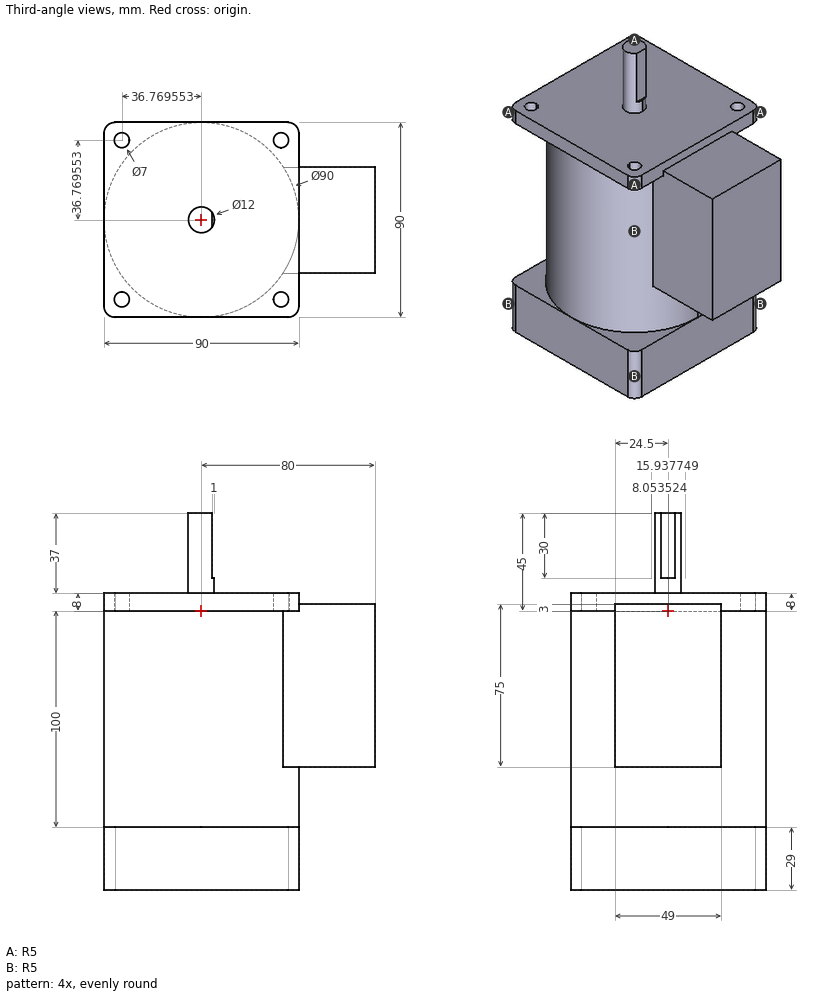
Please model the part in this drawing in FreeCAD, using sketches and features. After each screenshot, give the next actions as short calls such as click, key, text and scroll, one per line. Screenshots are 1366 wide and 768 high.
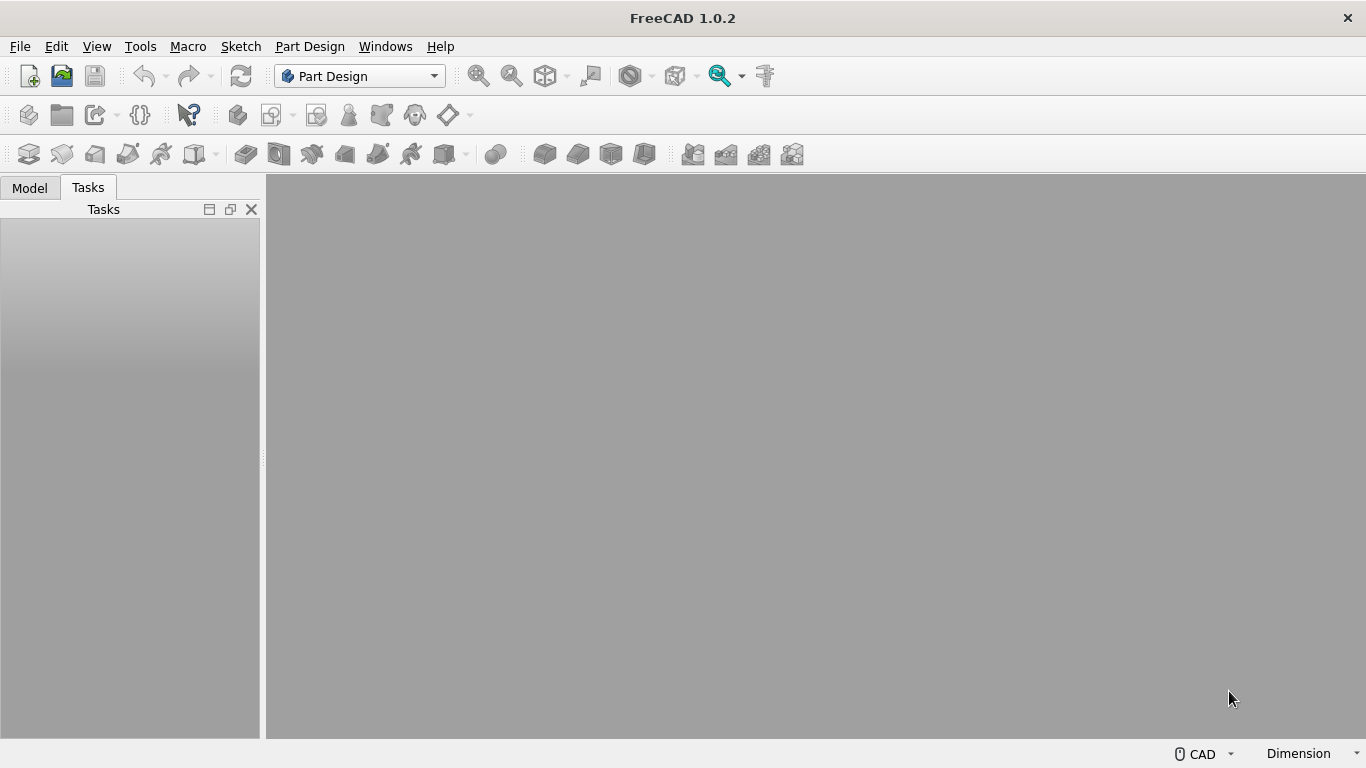
click(29, 76)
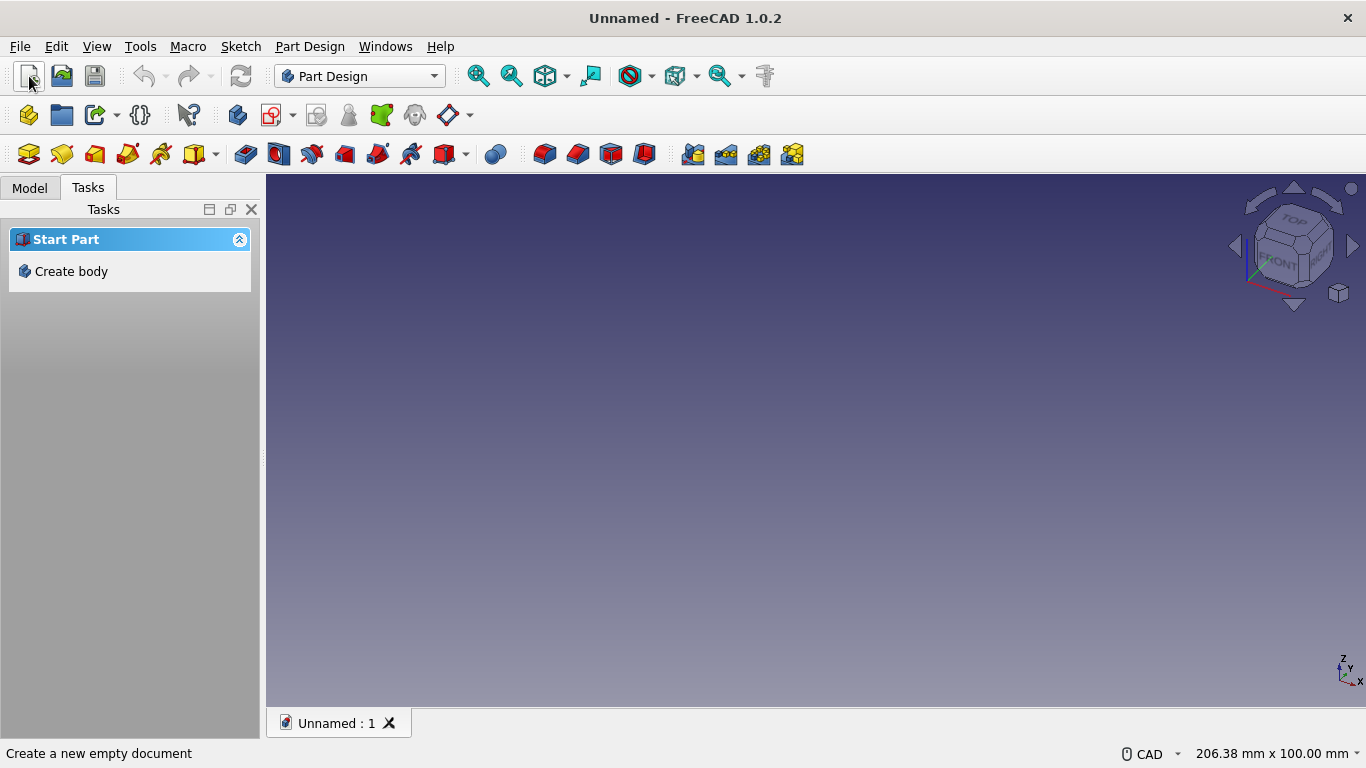
click(270, 116)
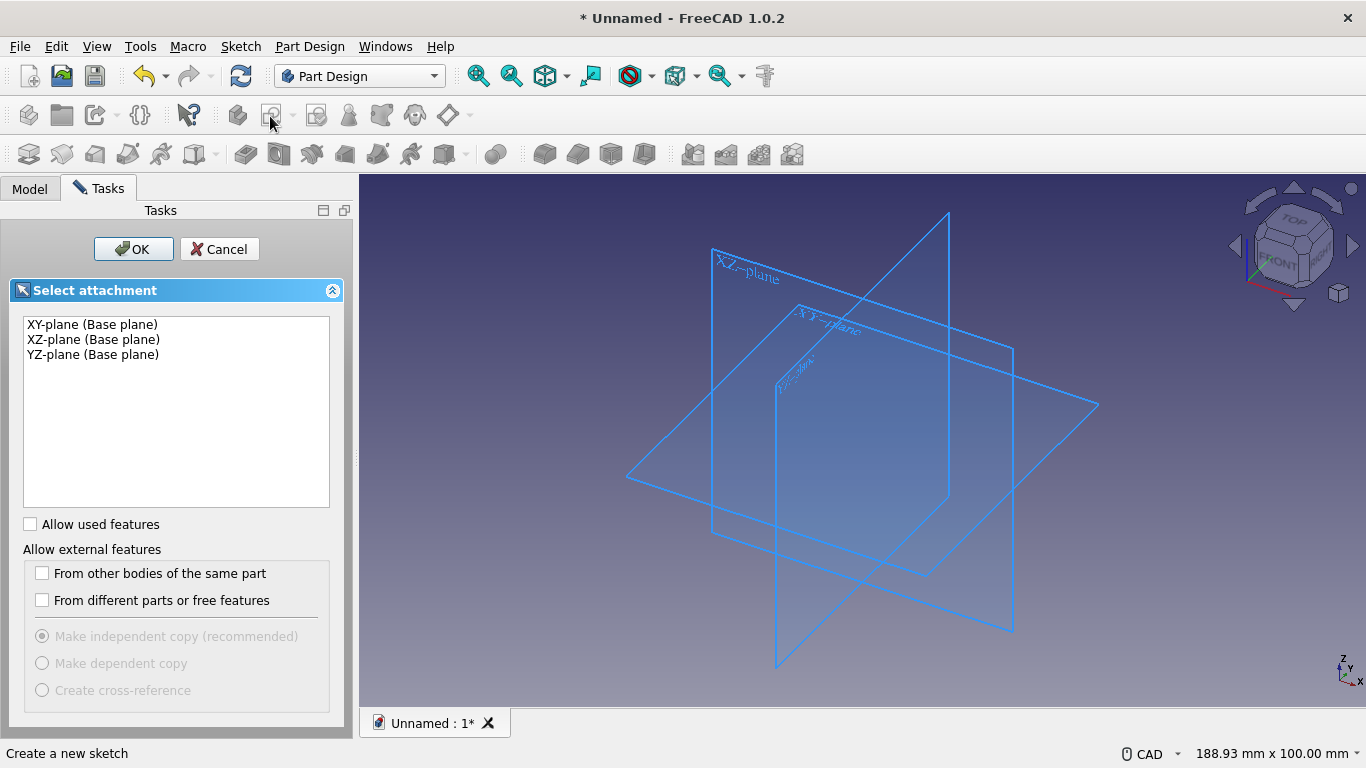
click(84, 324)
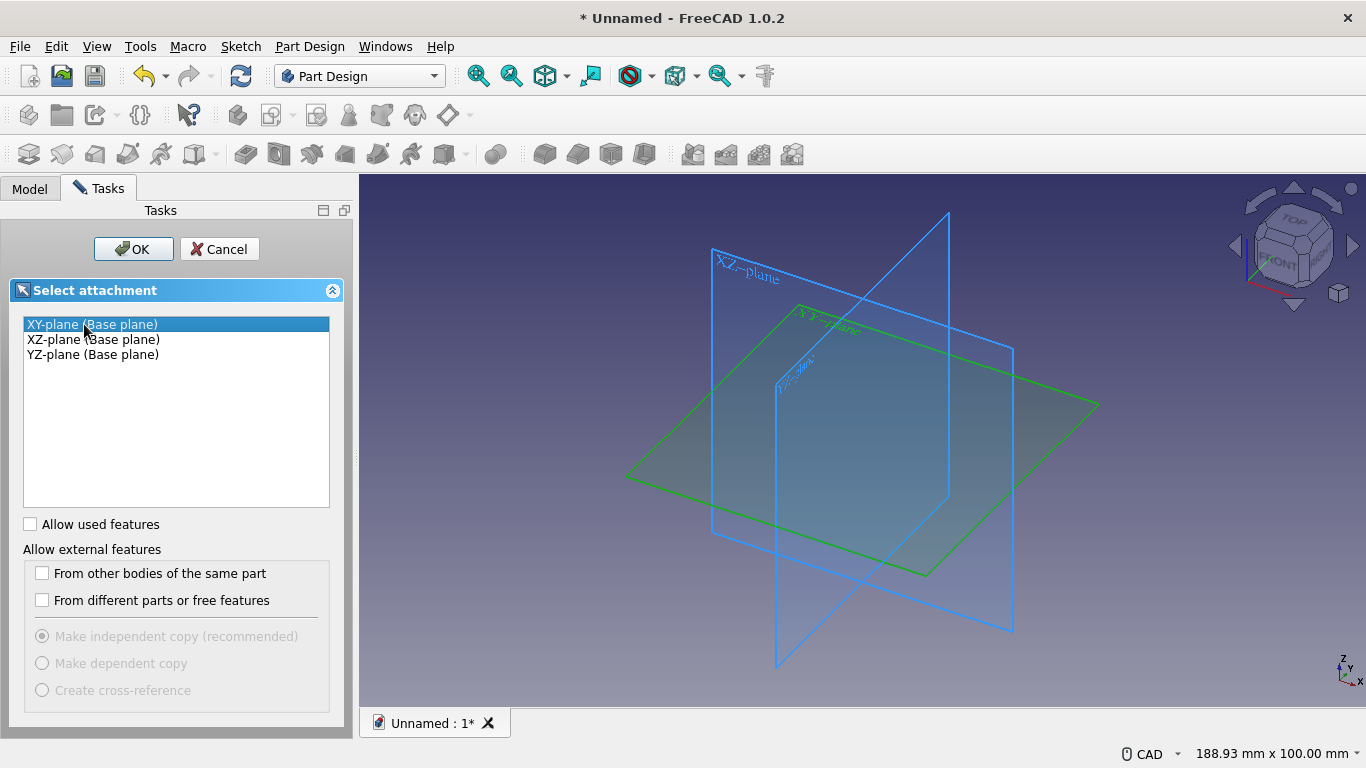
click(134, 249)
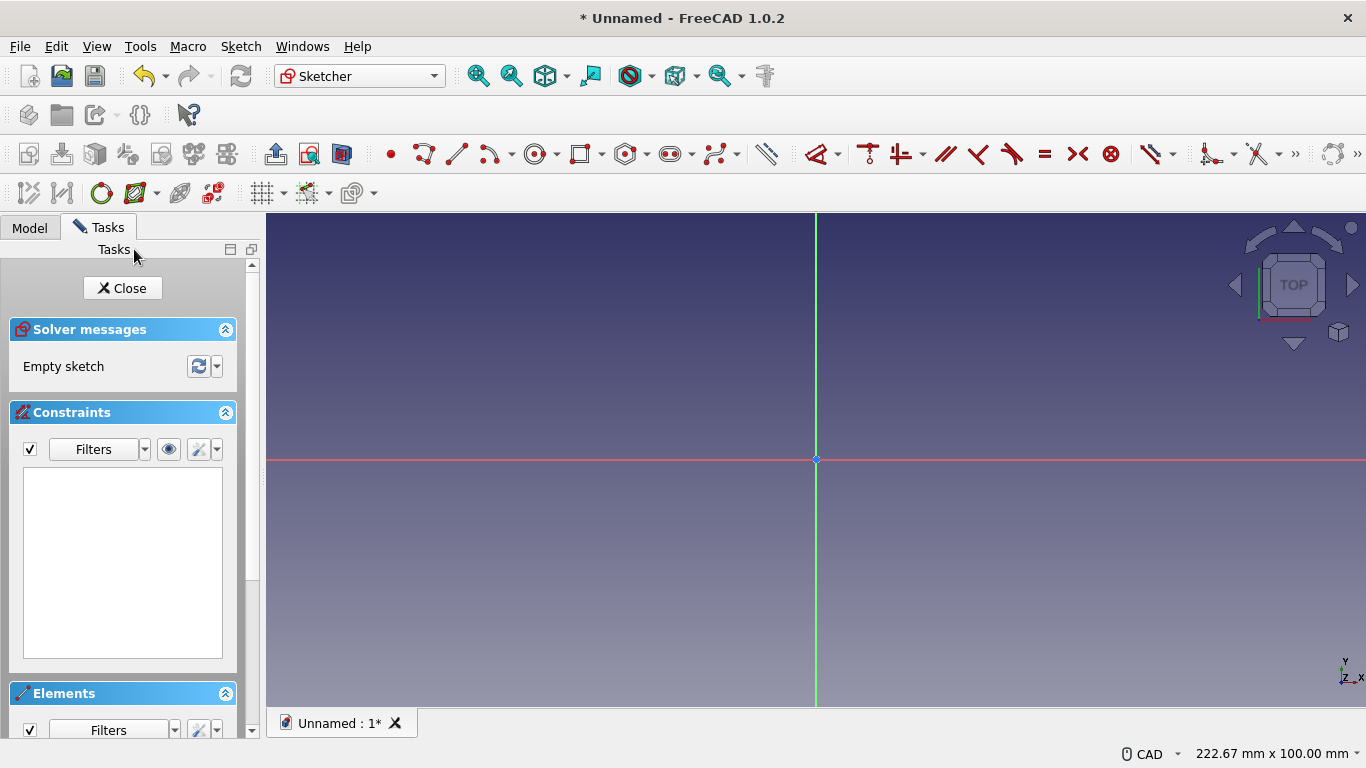
scroll(608, 460, down, 2)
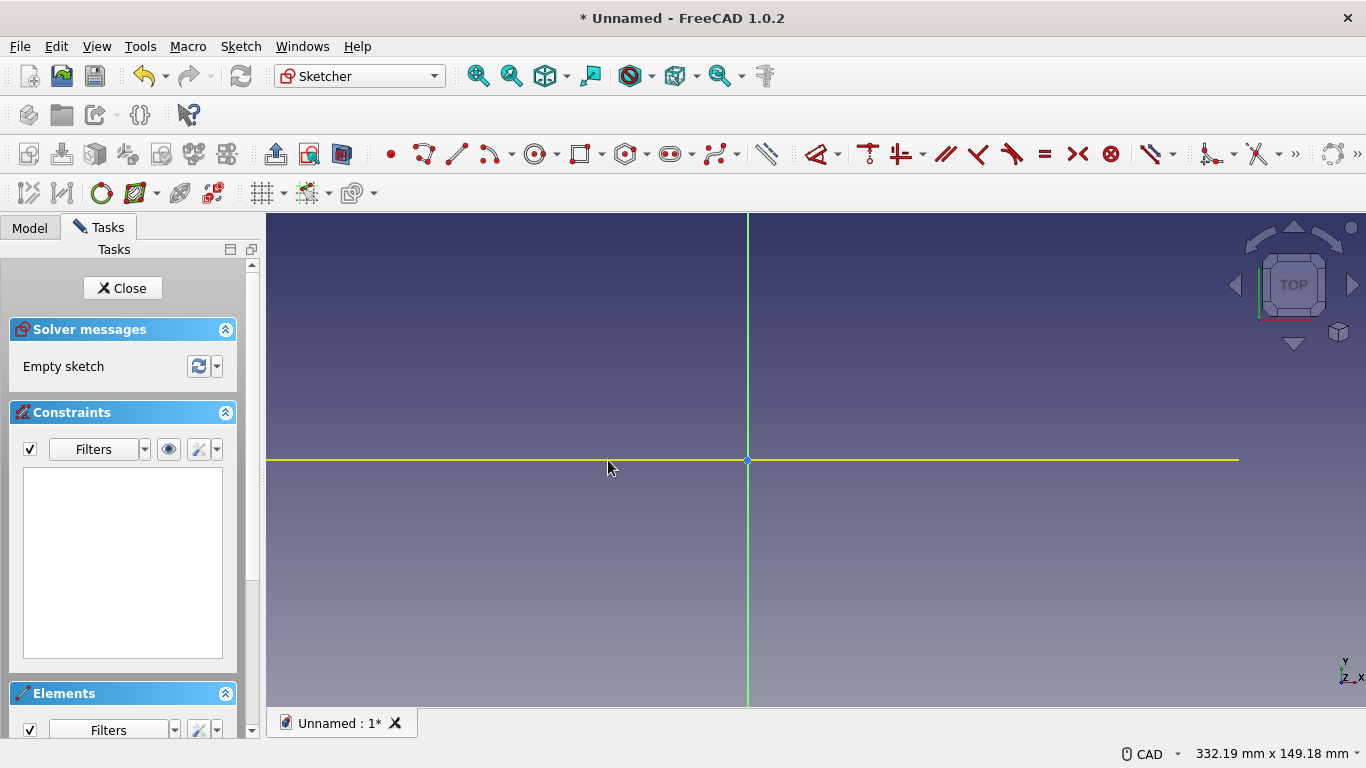
key(g)
key(v)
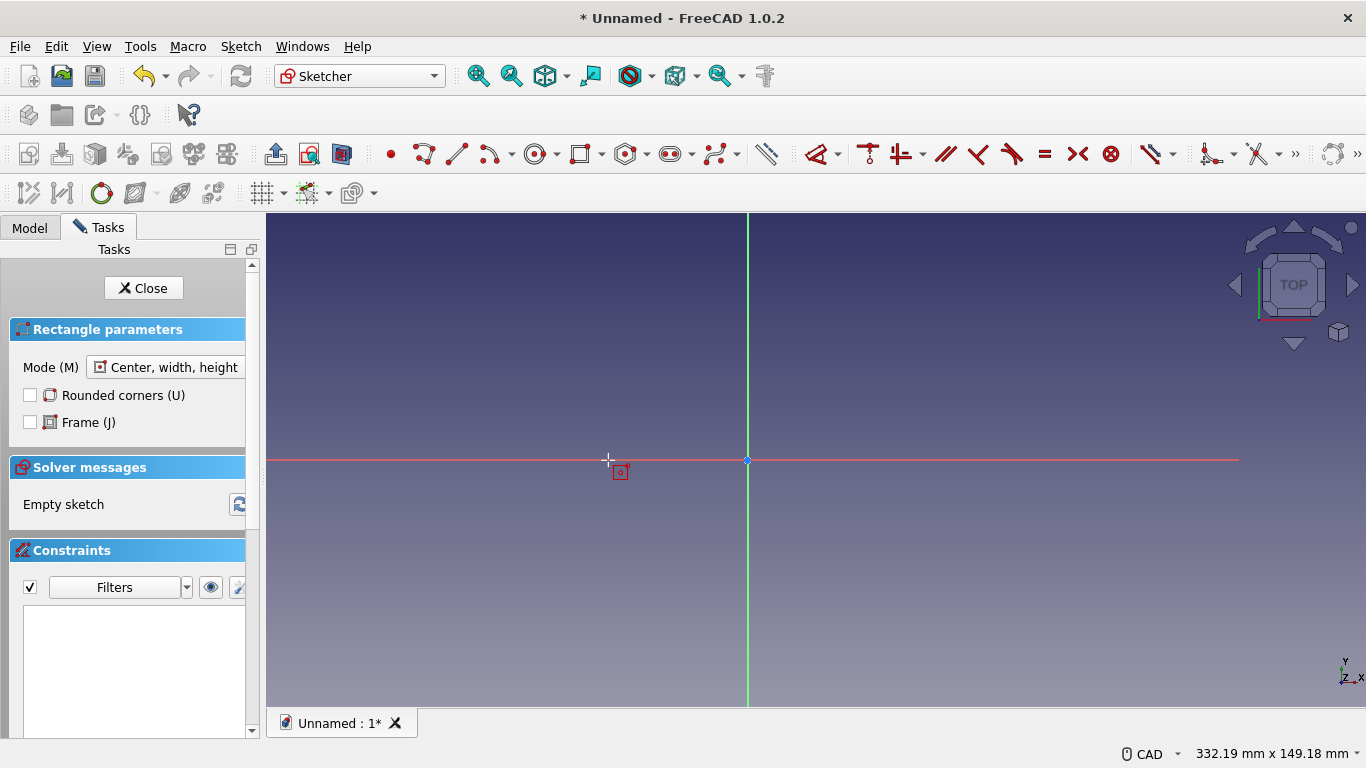
click(748, 460)
click(897, 311)
key(Escape)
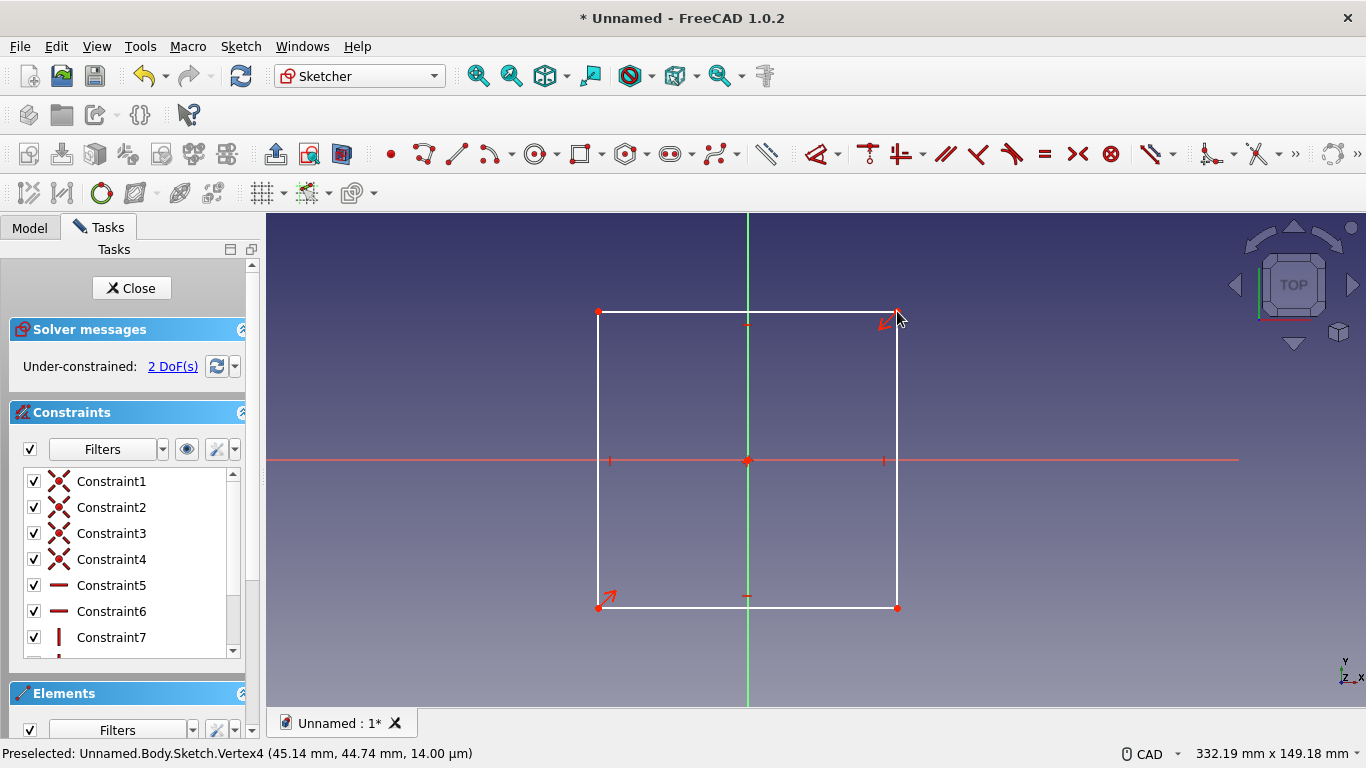
click(688, 608)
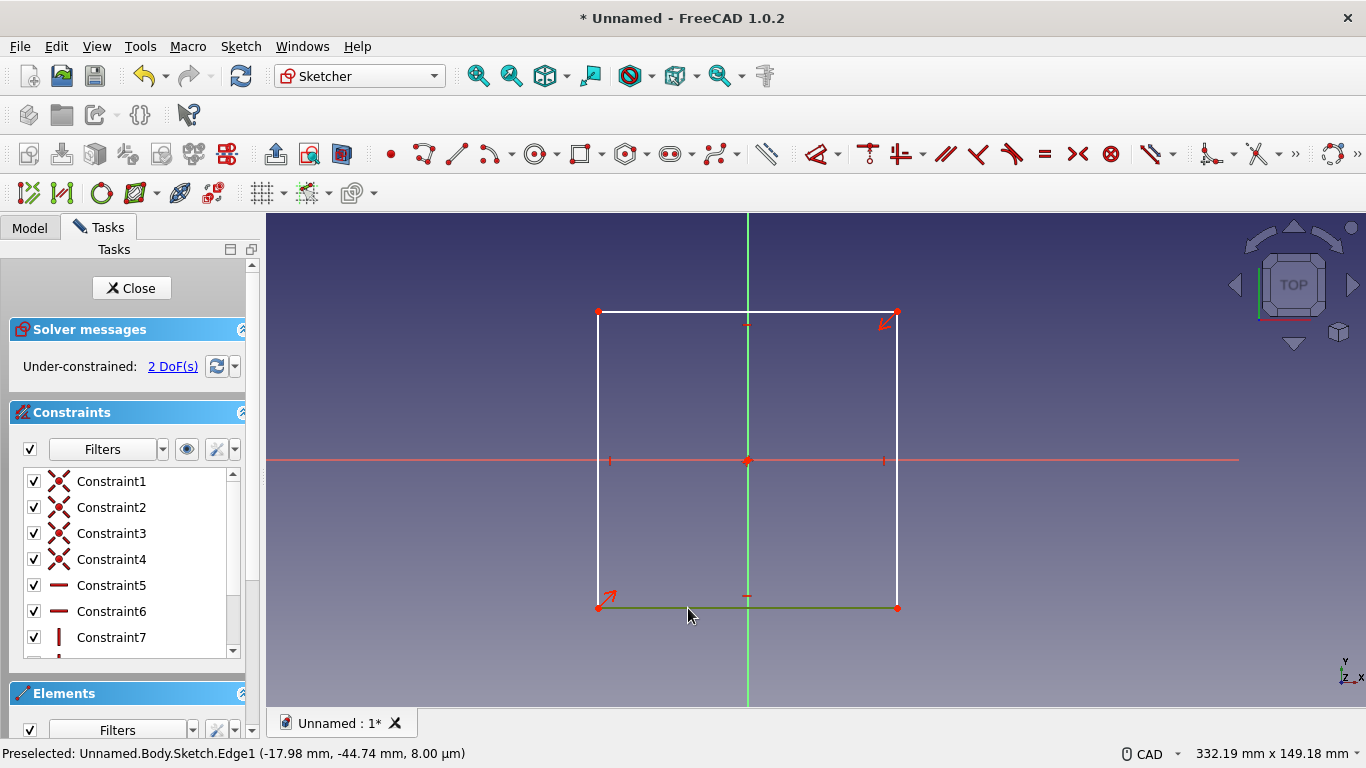
click(838, 154)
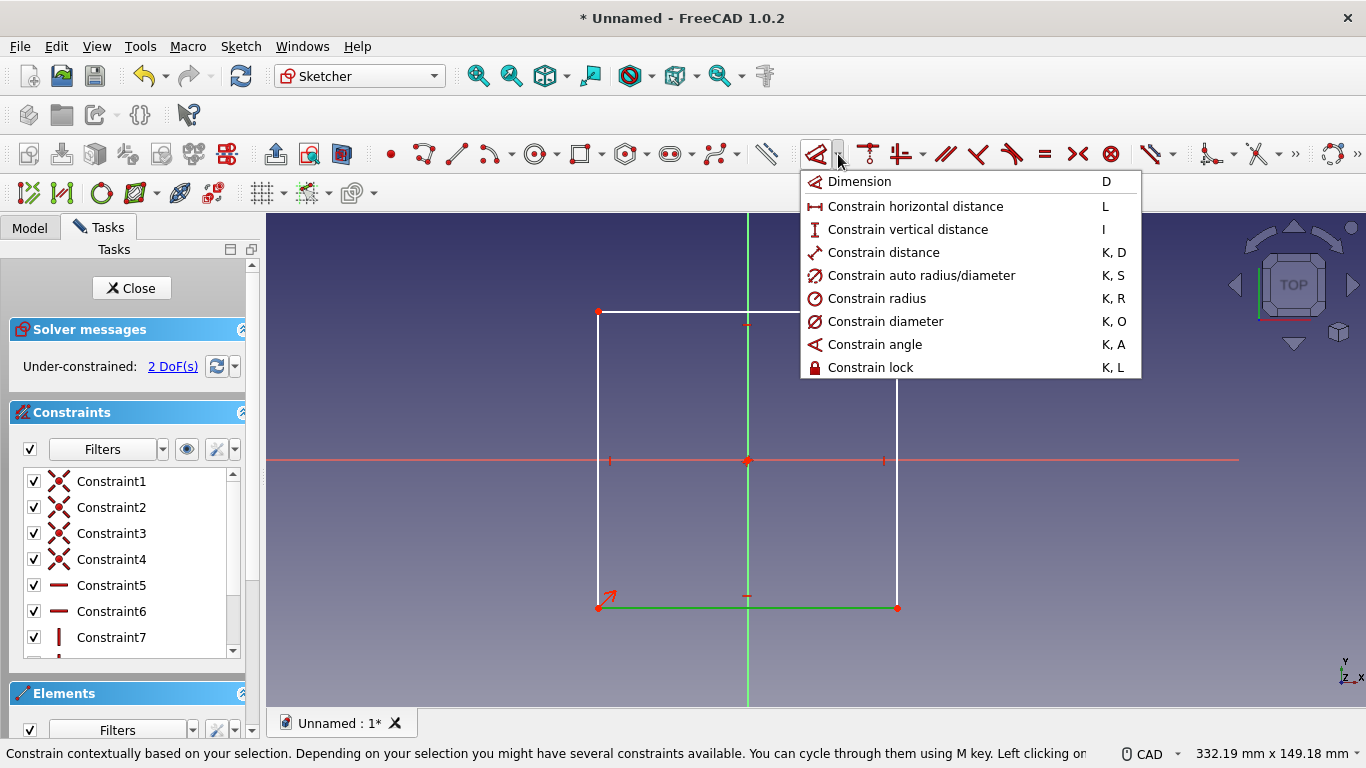
click(971, 206)